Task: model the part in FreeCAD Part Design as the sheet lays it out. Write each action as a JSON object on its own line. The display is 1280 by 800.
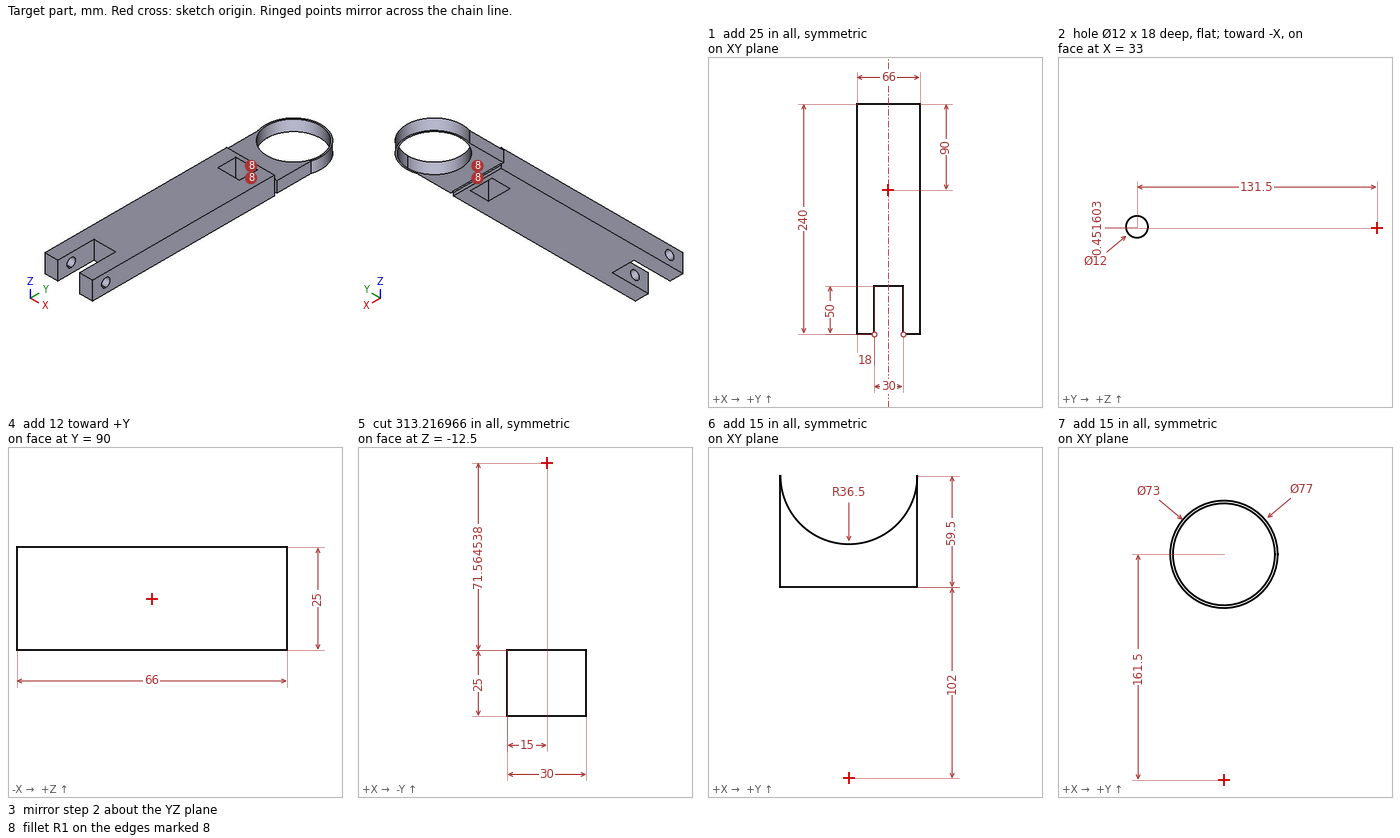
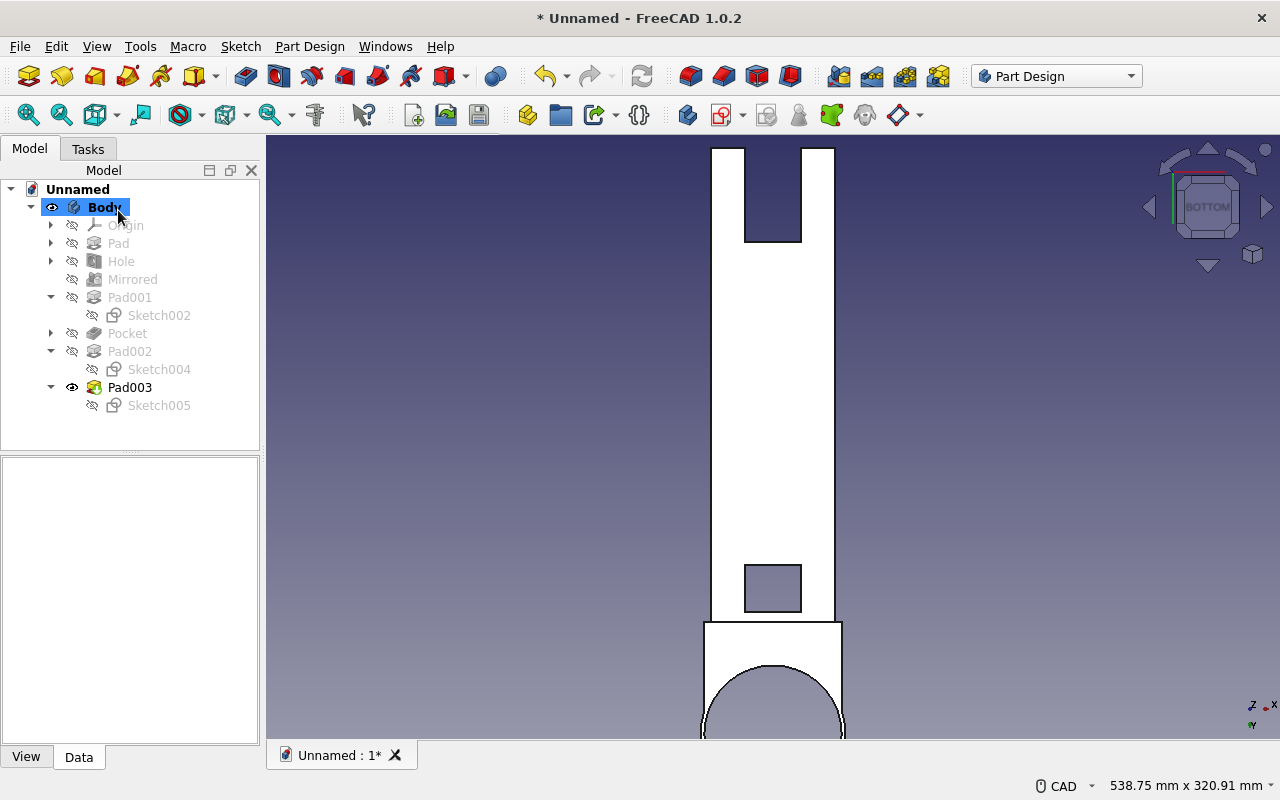
{"action": "left_click", "coordinate": [29, 116]}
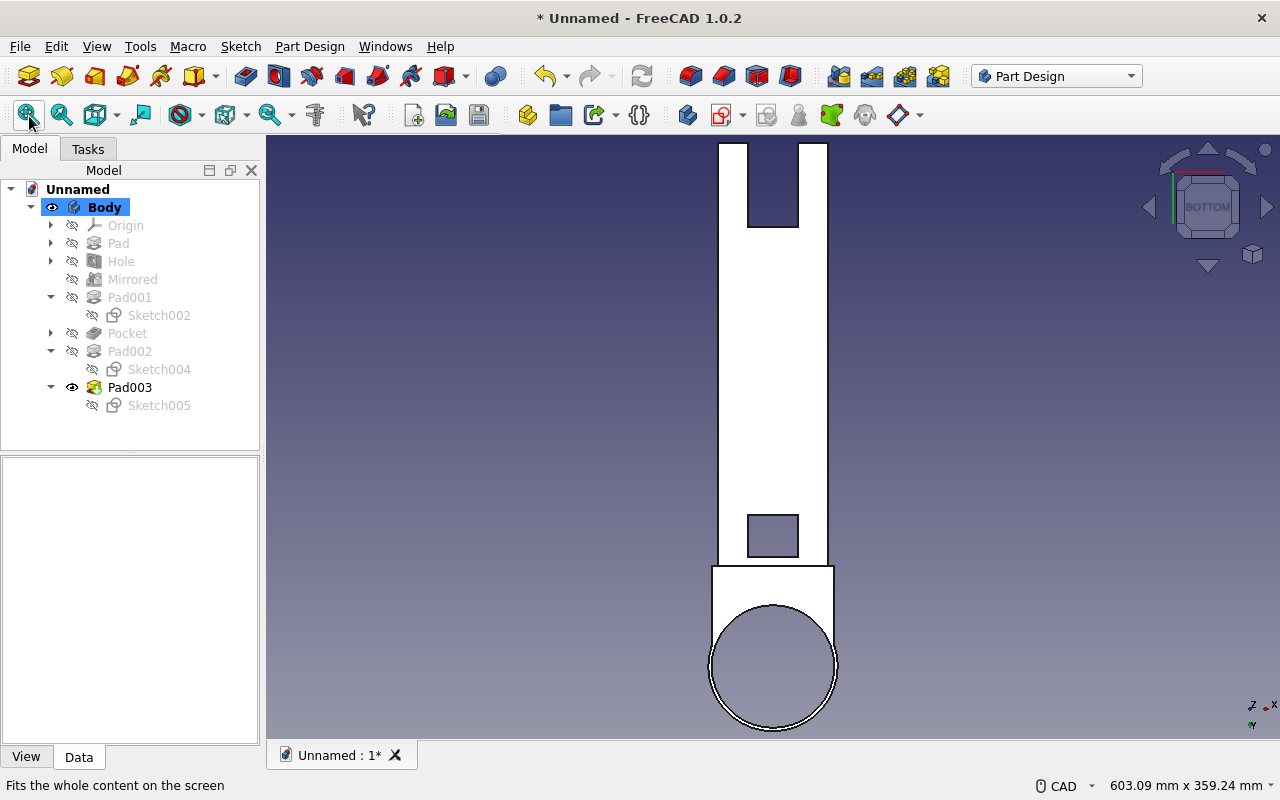
{"action": "key", "text": "0"}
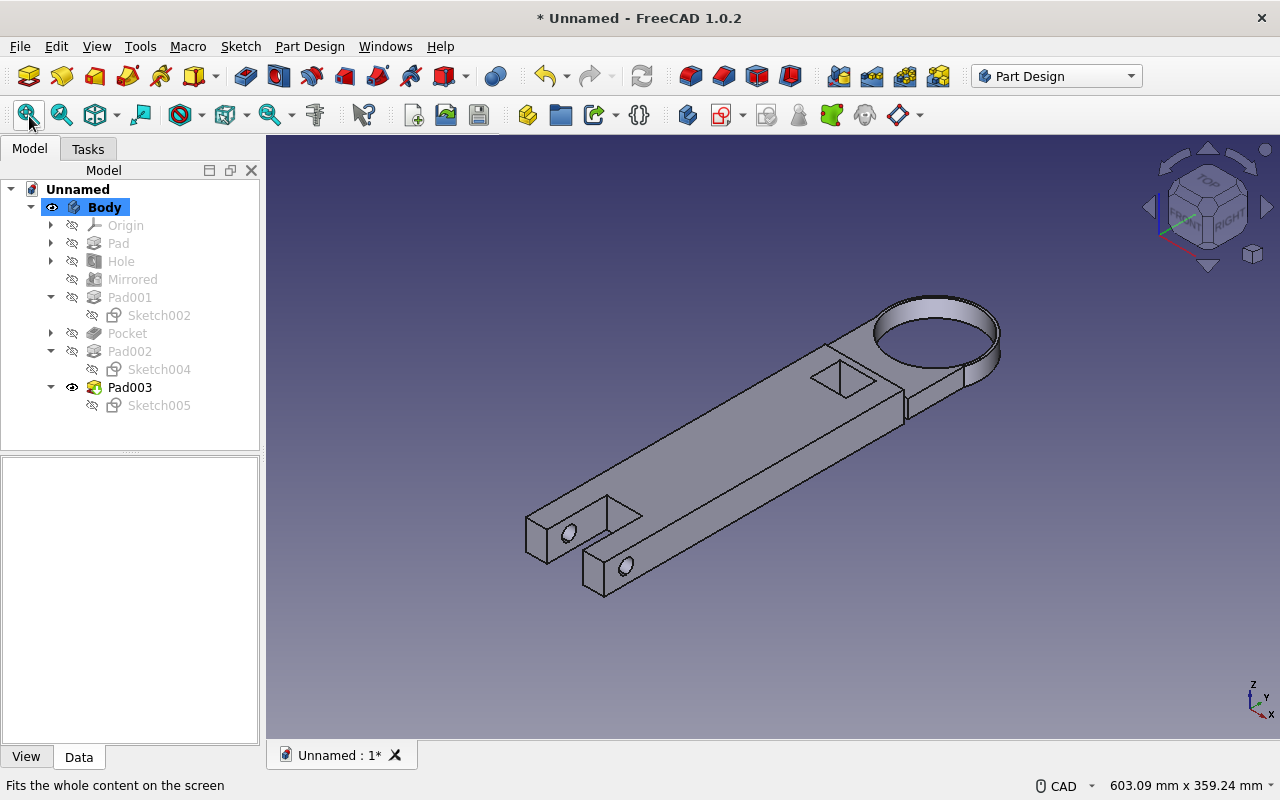
{"action": "key", "text": "2"}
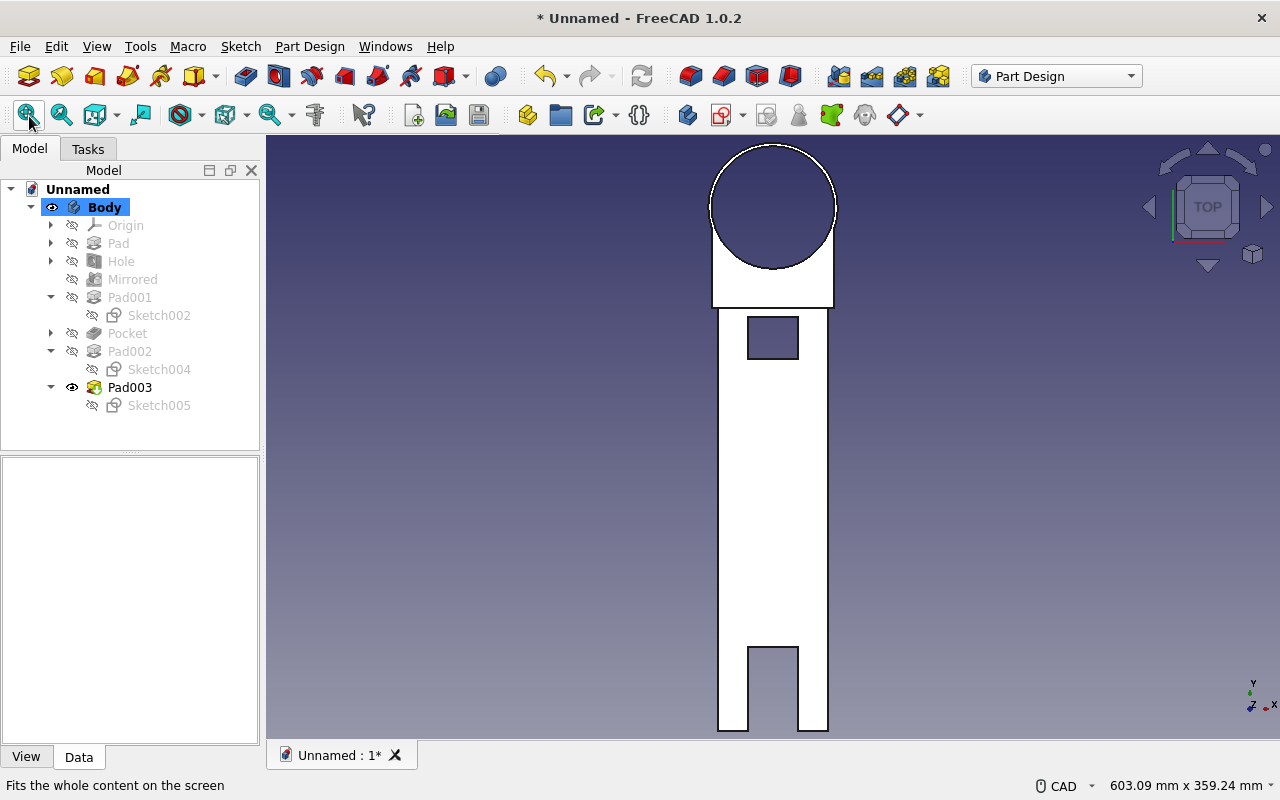
{"action": "key", "text": "1"}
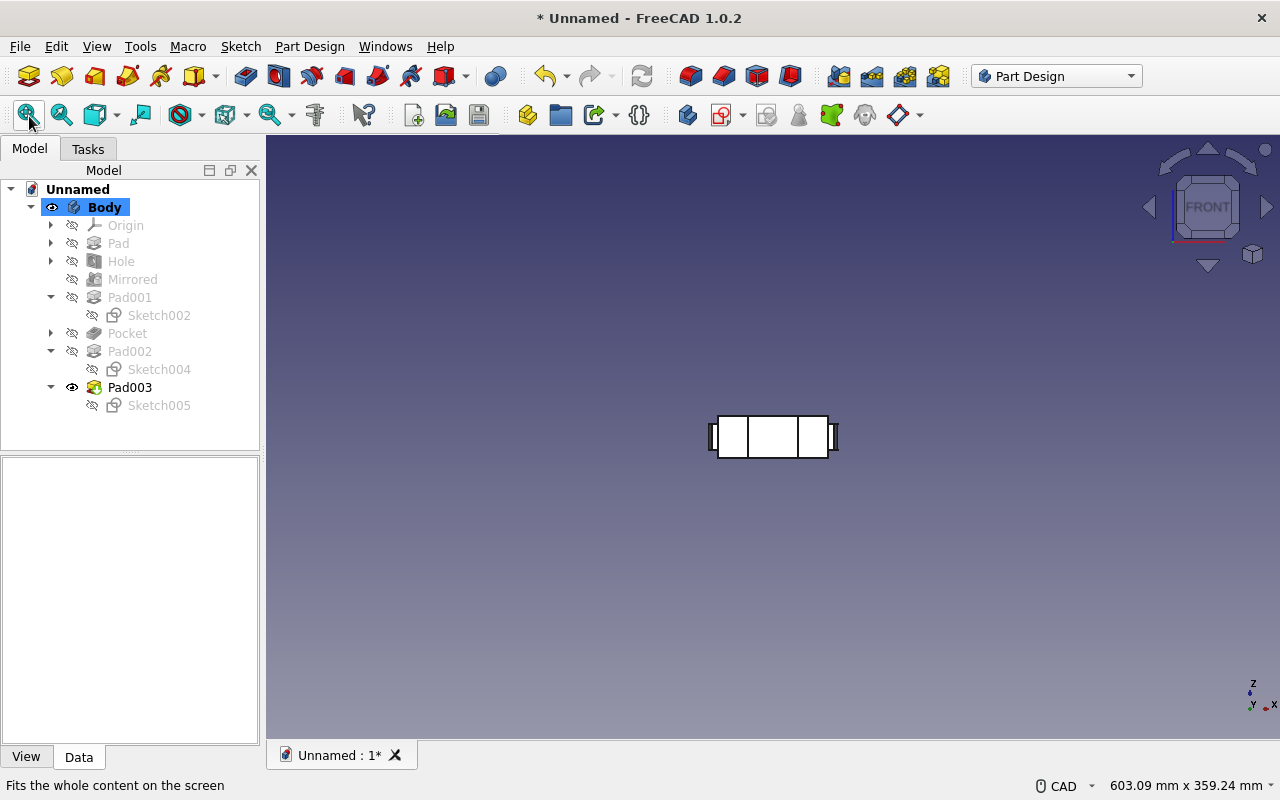
{"action": "left_click", "coordinate": [29, 116]}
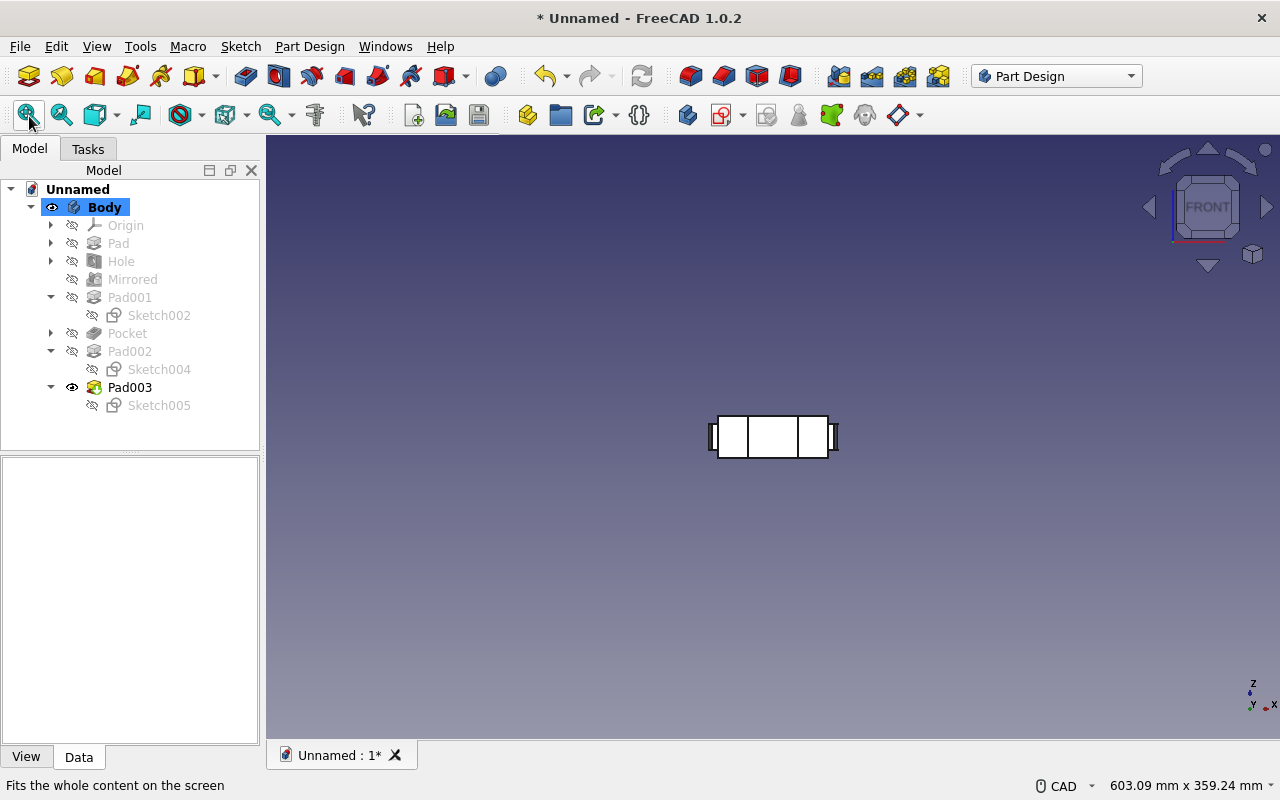
{"action": "key", "text": "3"}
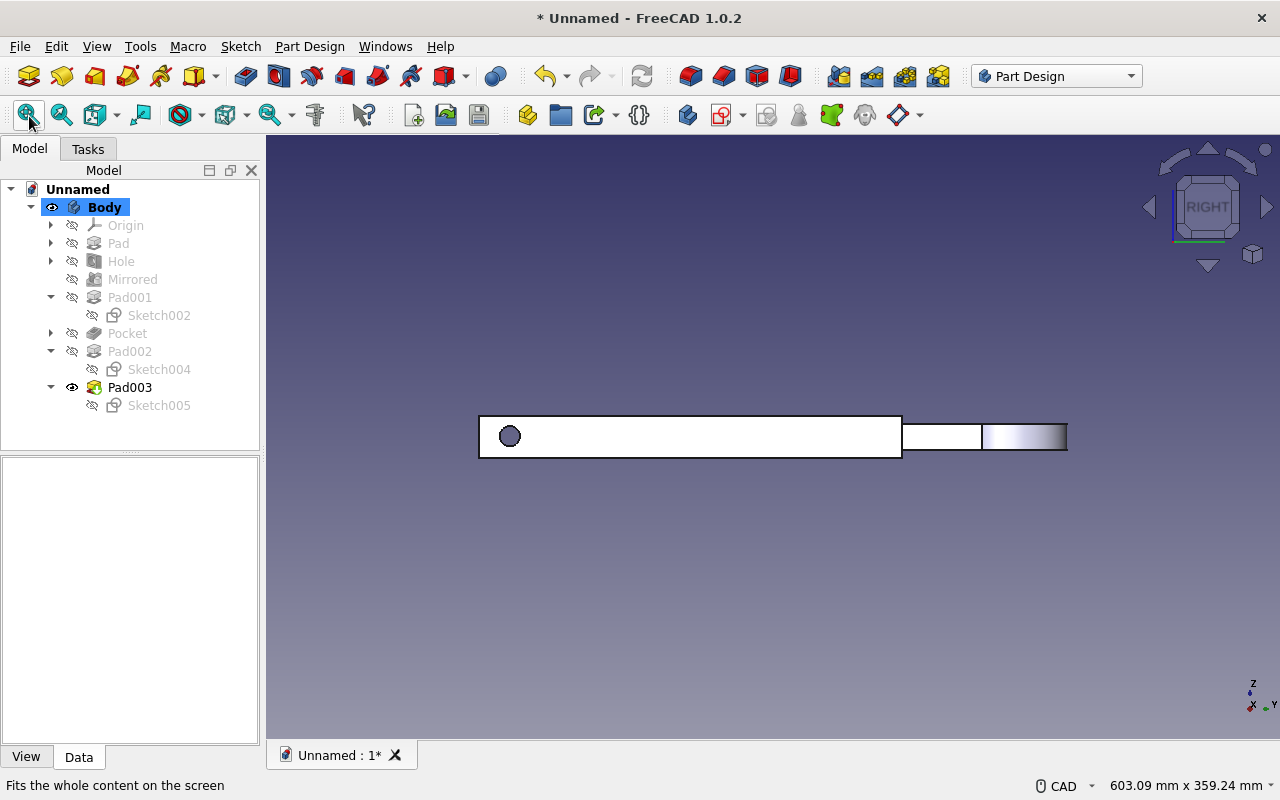
{"action": "key", "text": "5"}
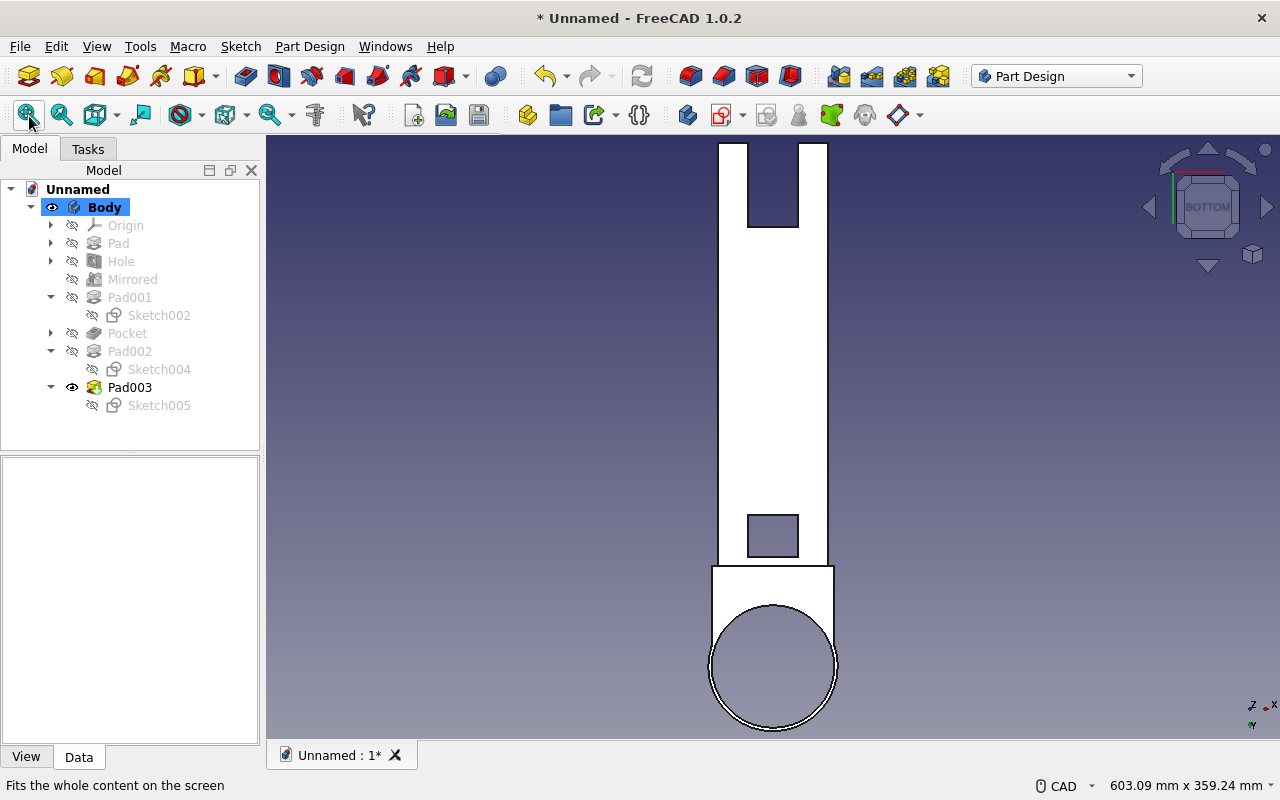
{"action": "key", "text": "4"}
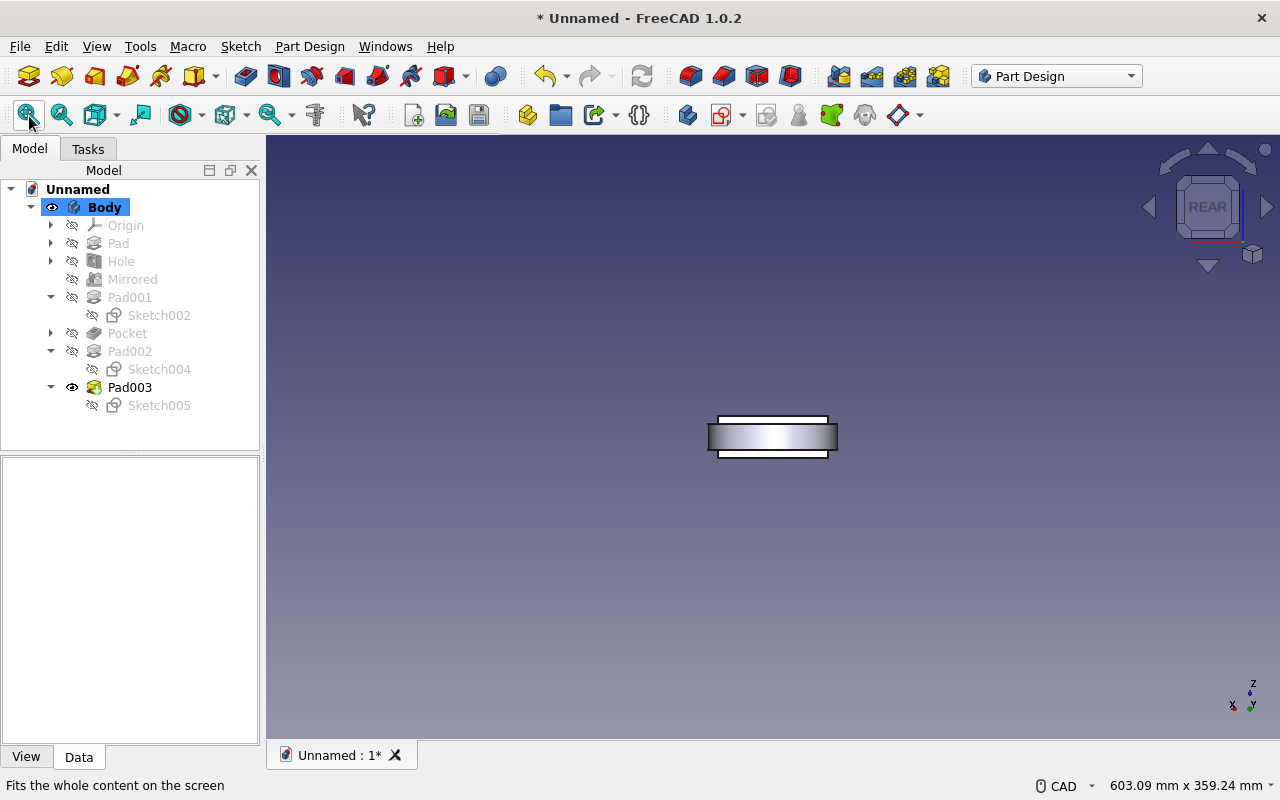
{"action": "key", "text": "v f"}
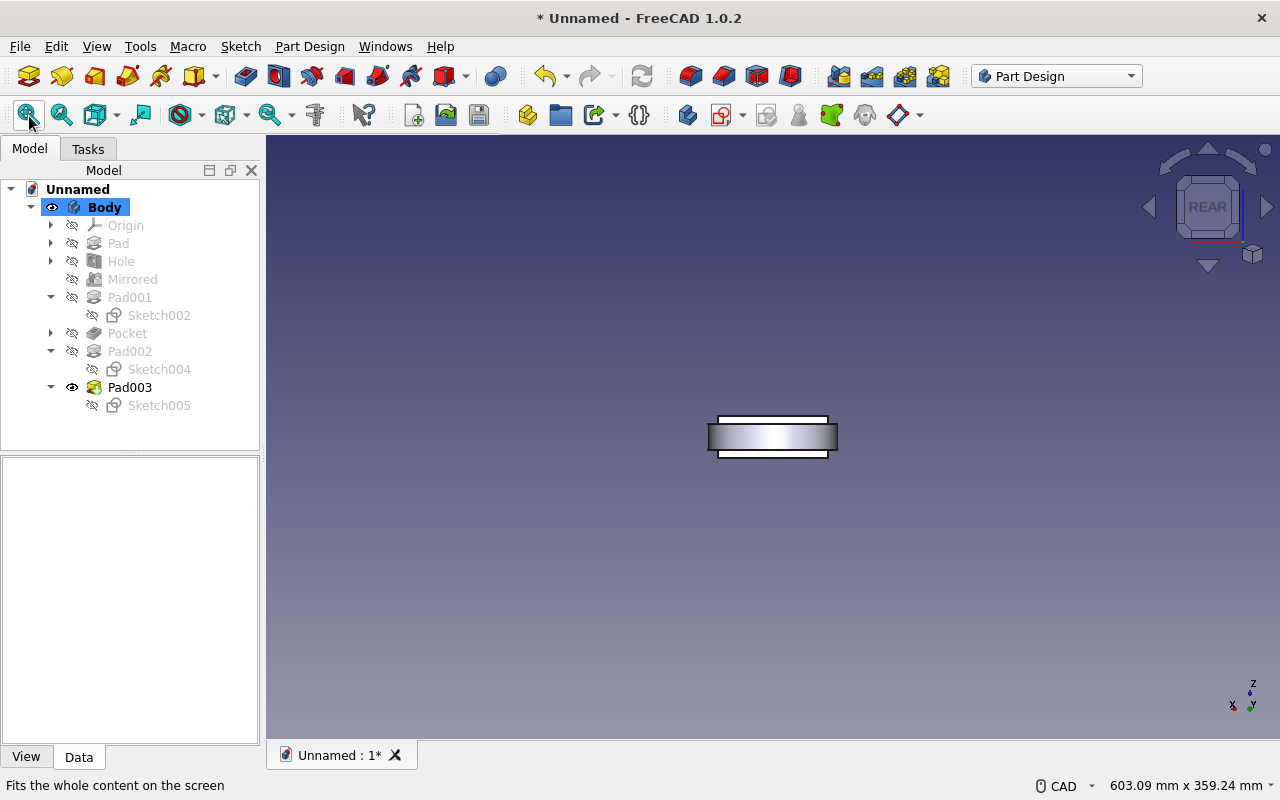
{"action": "key", "text": "6"}